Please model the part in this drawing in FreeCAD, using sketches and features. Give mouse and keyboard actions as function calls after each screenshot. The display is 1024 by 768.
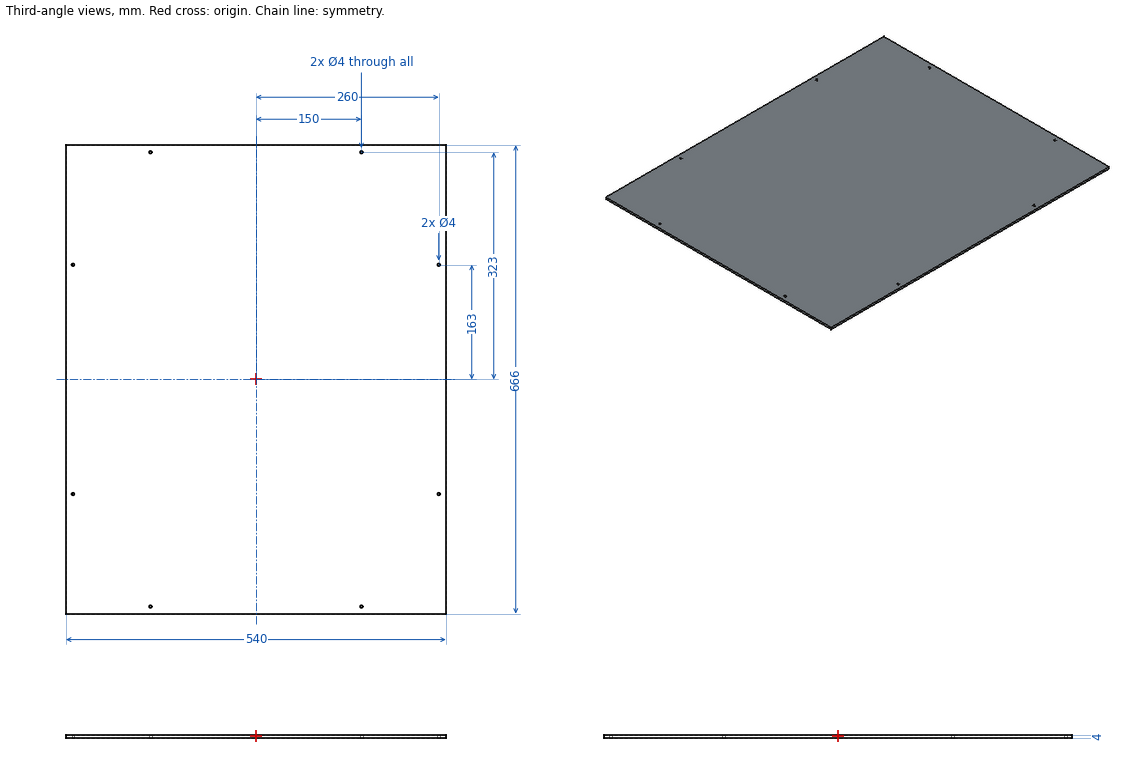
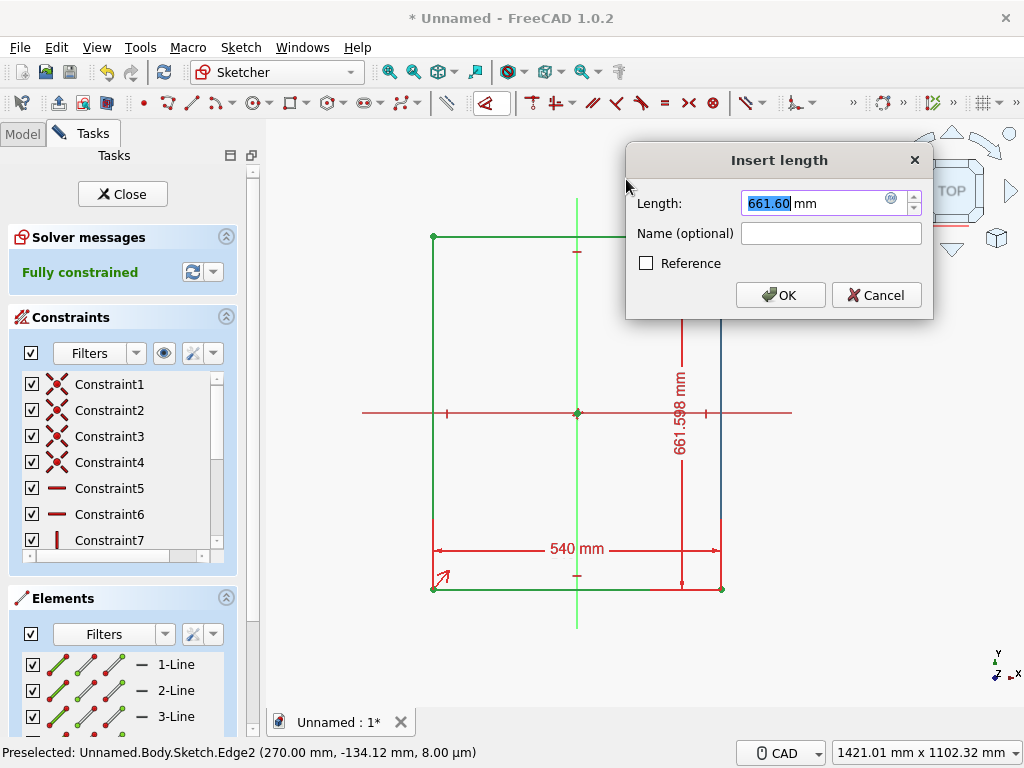
text(666)
key(Return)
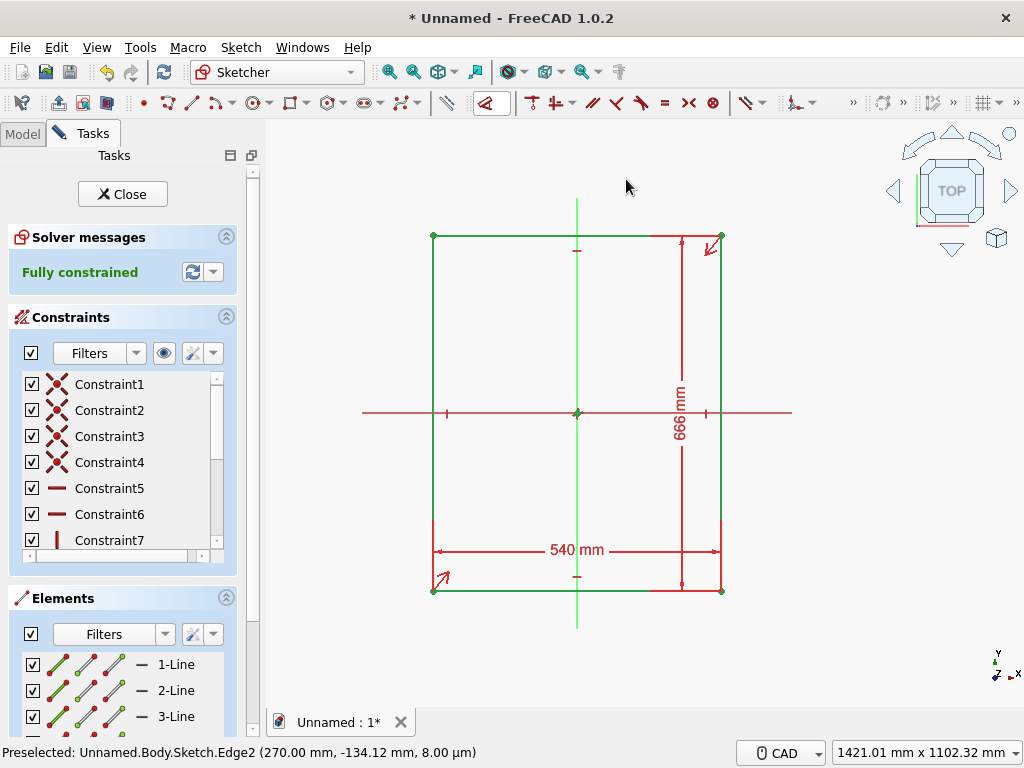
click(123, 194)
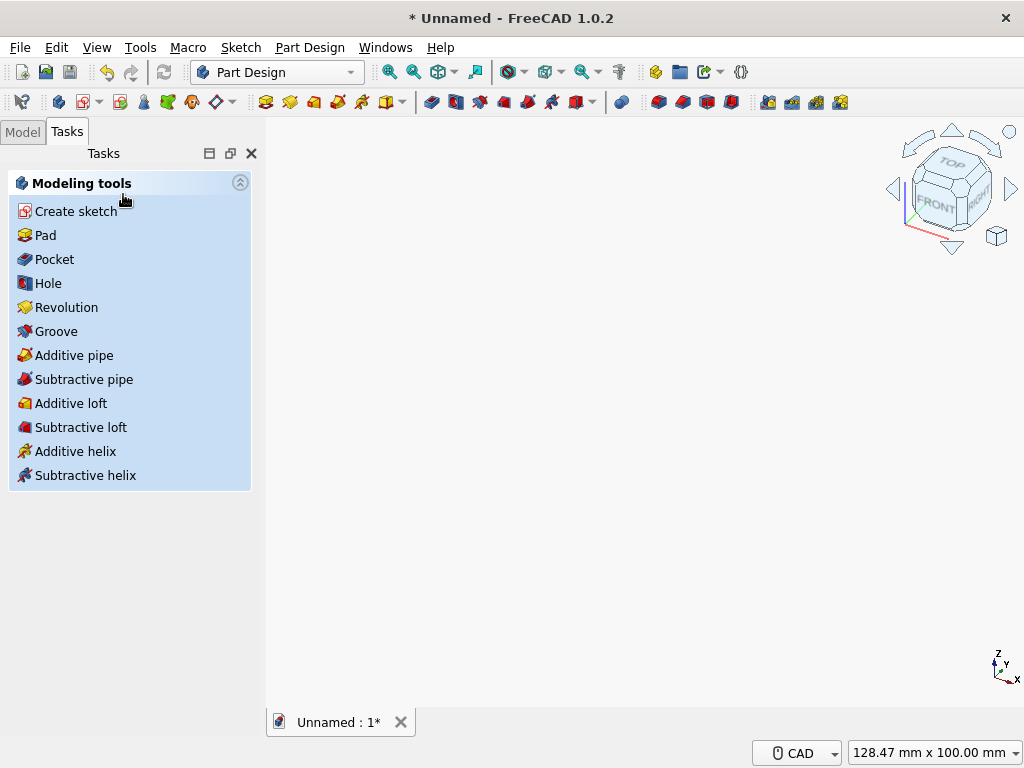
click(266, 102)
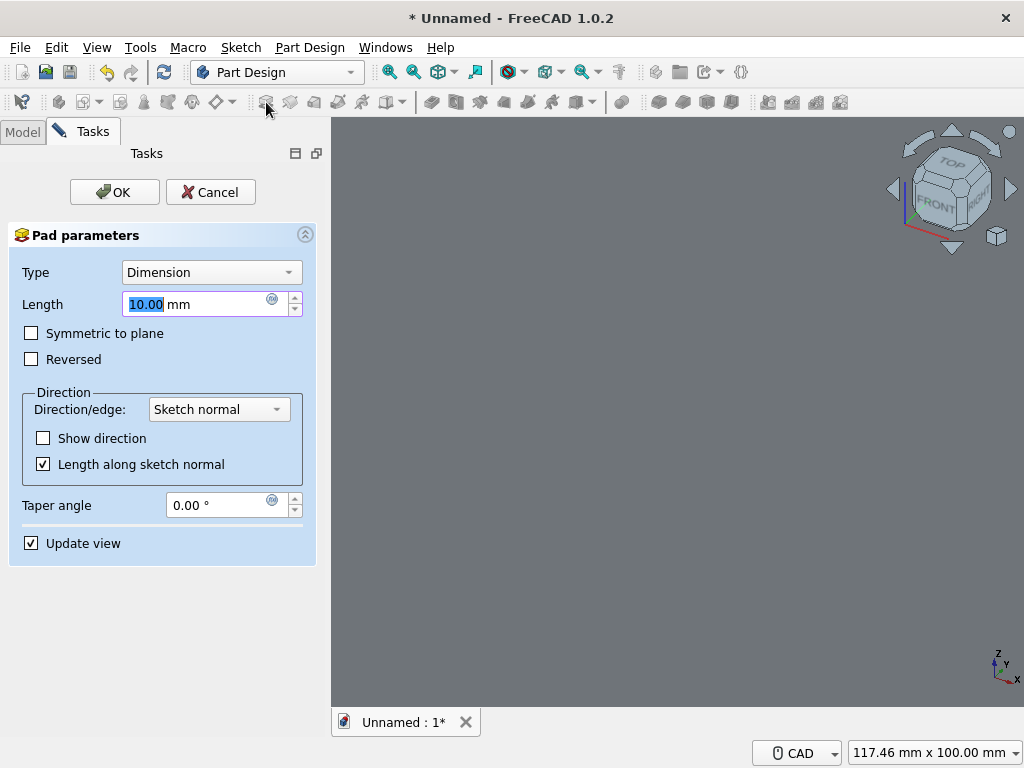
text(4)
key(Tab)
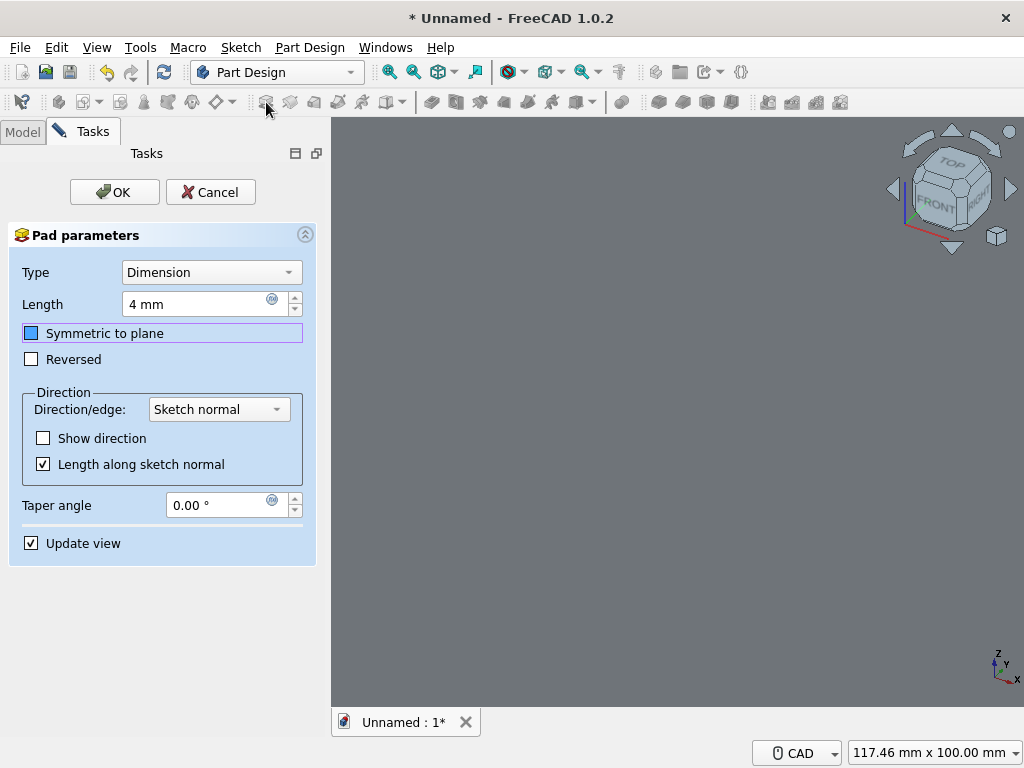
click(30, 333)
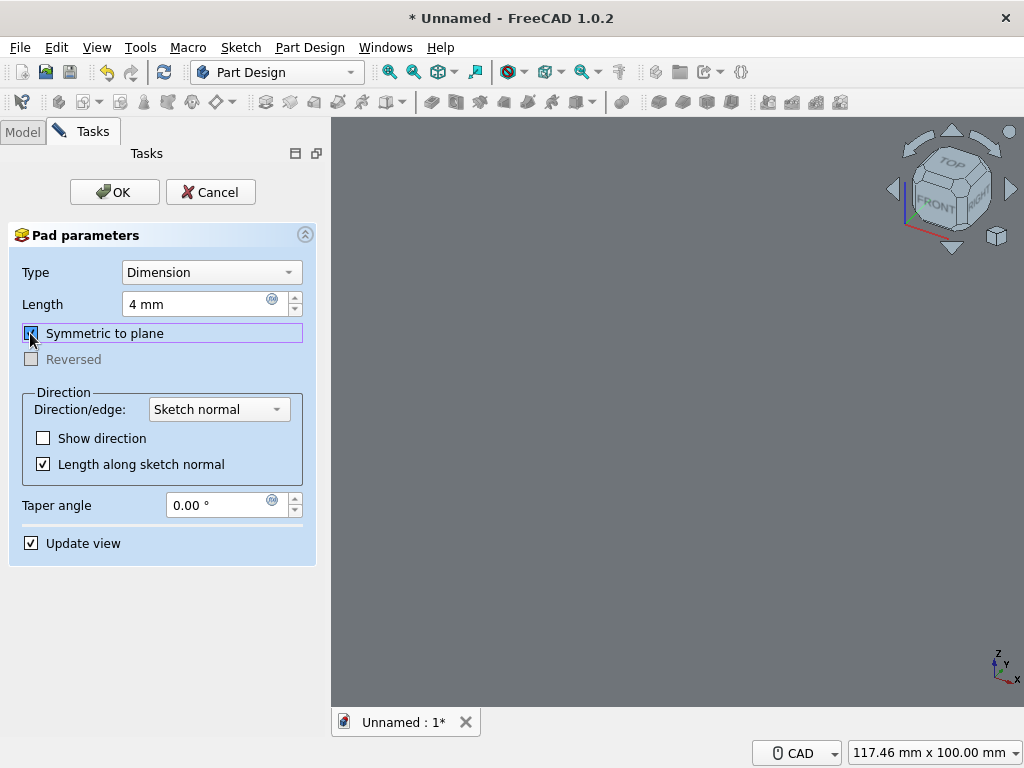
click(115, 192)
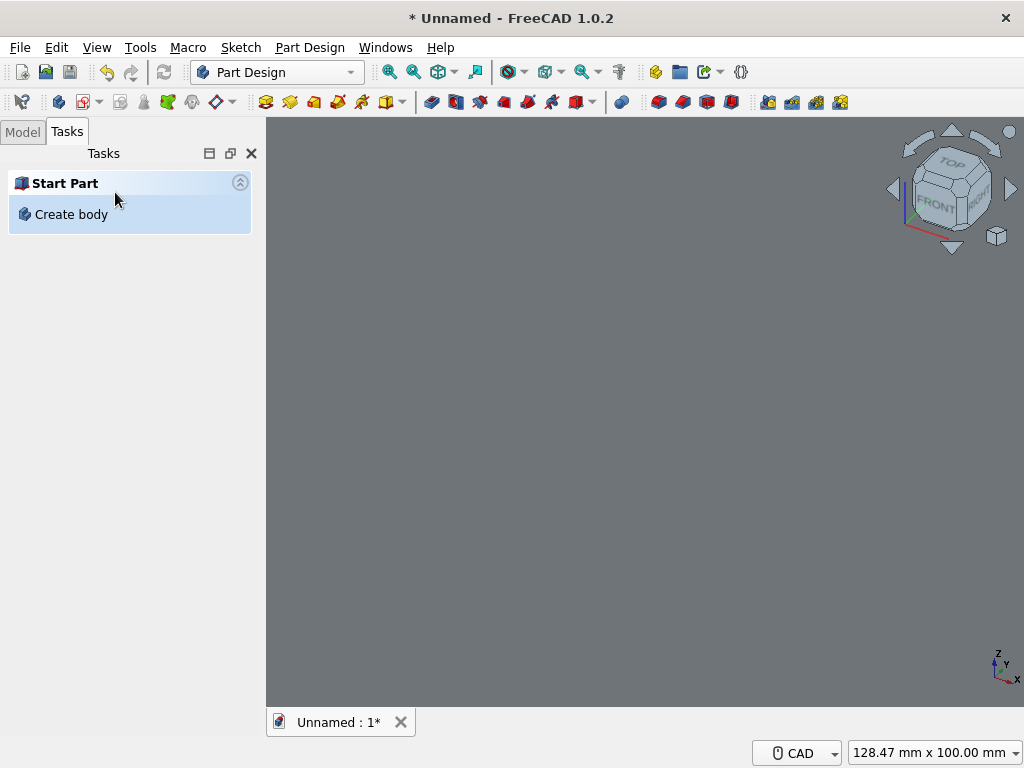
key(v)
key(f)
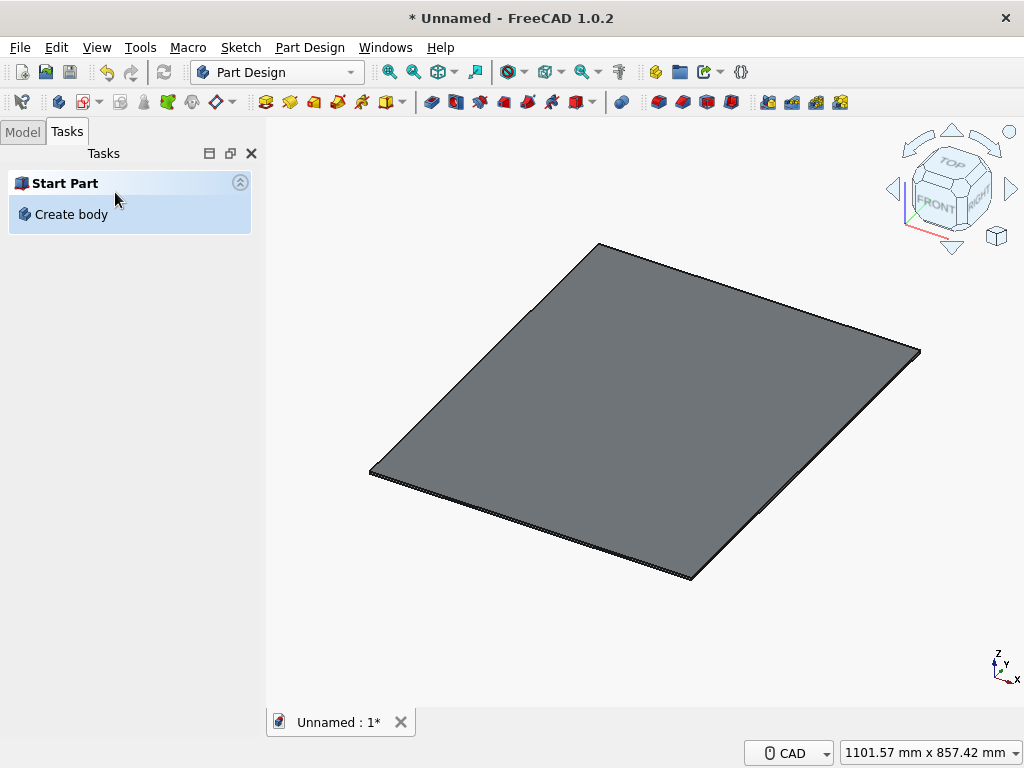
key(5)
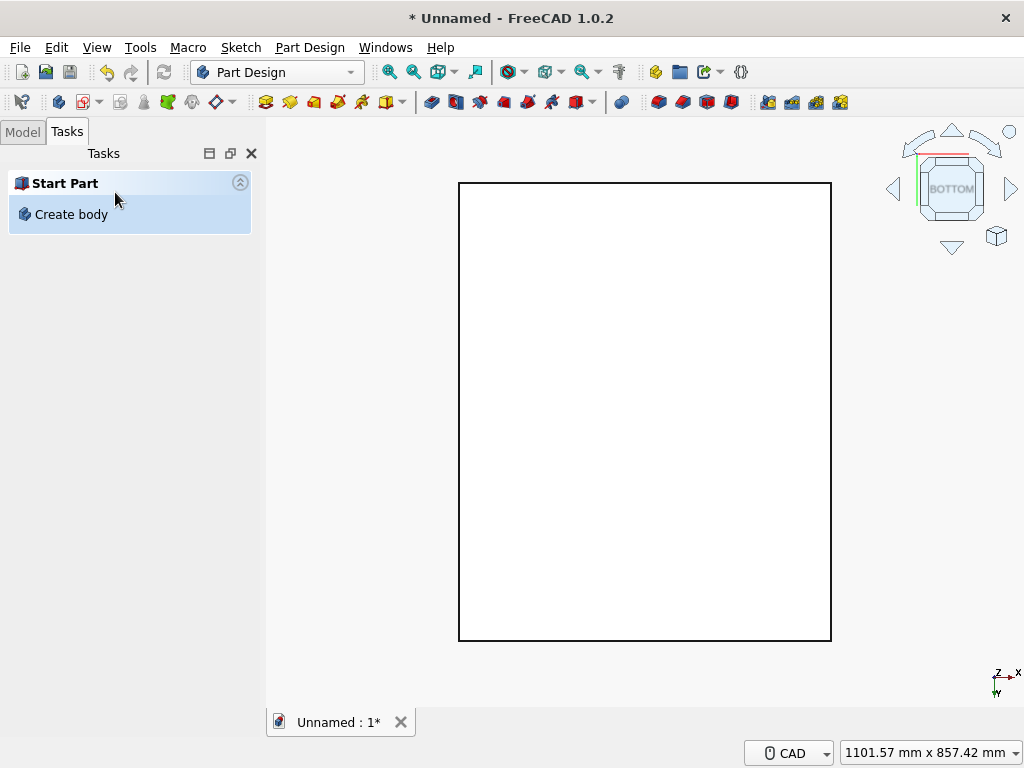
click(645, 411)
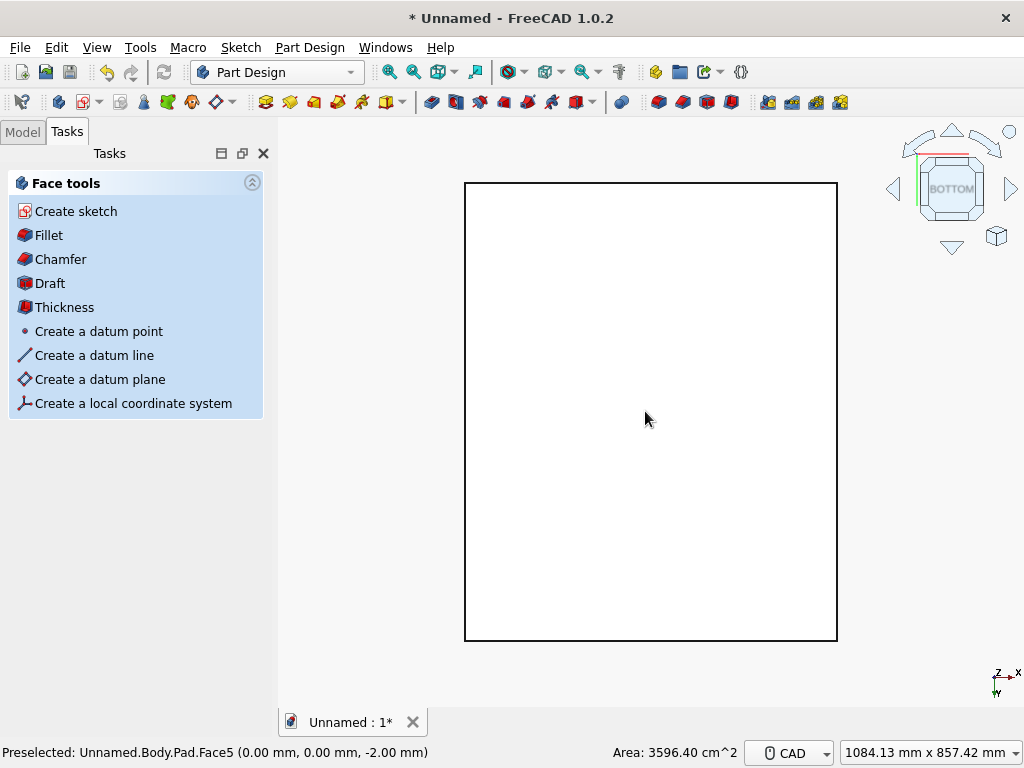
click(84, 102)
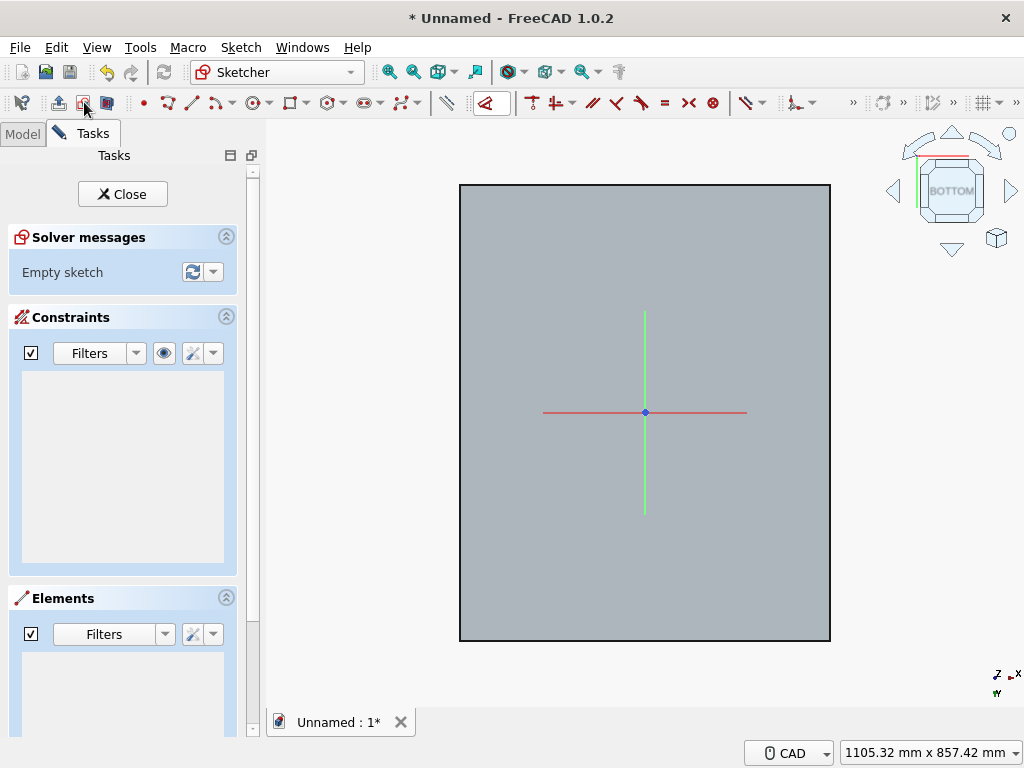
scroll(859, 413, up, 3)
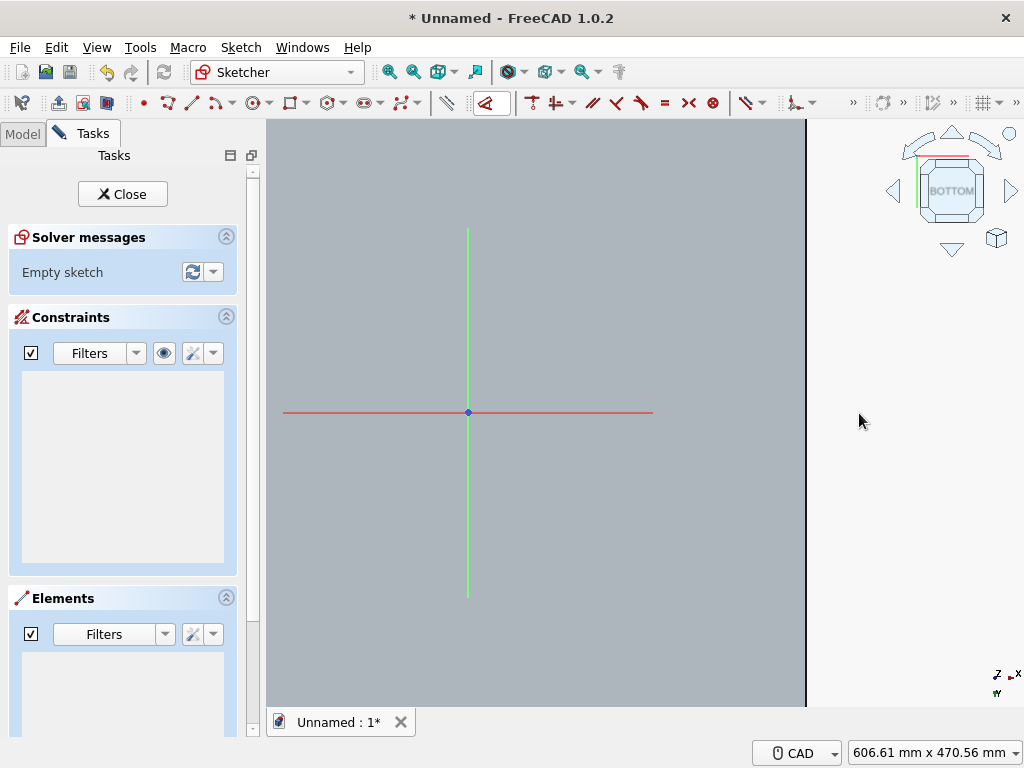
click(254, 104)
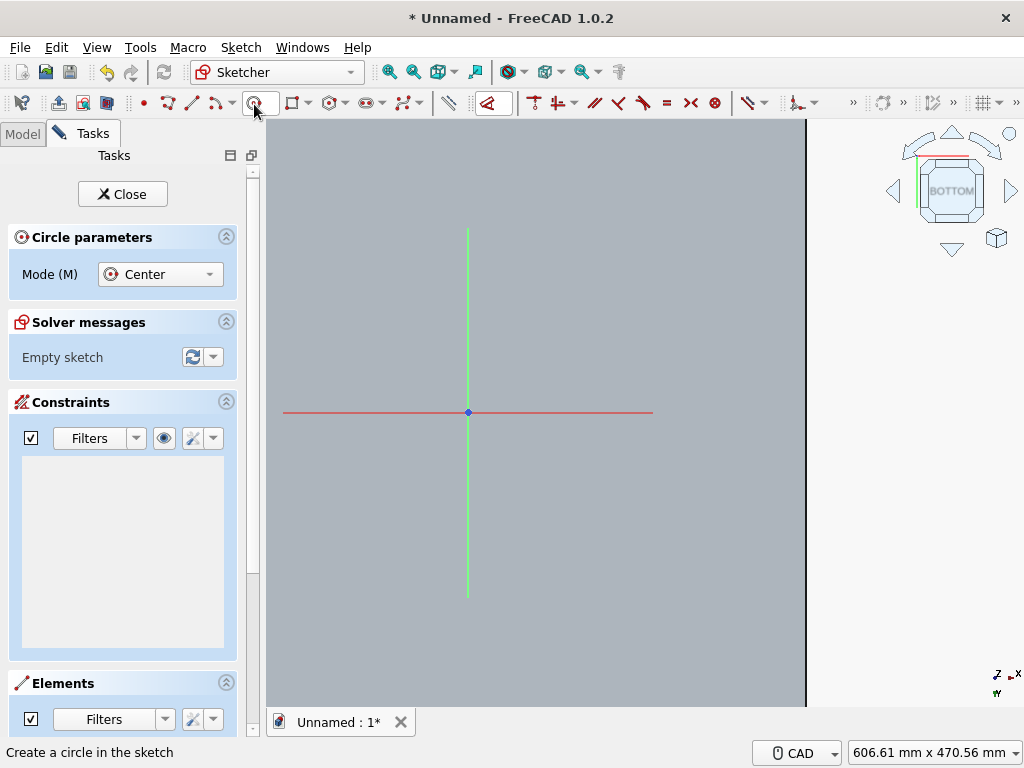
scroll(793, 616, up, 12)